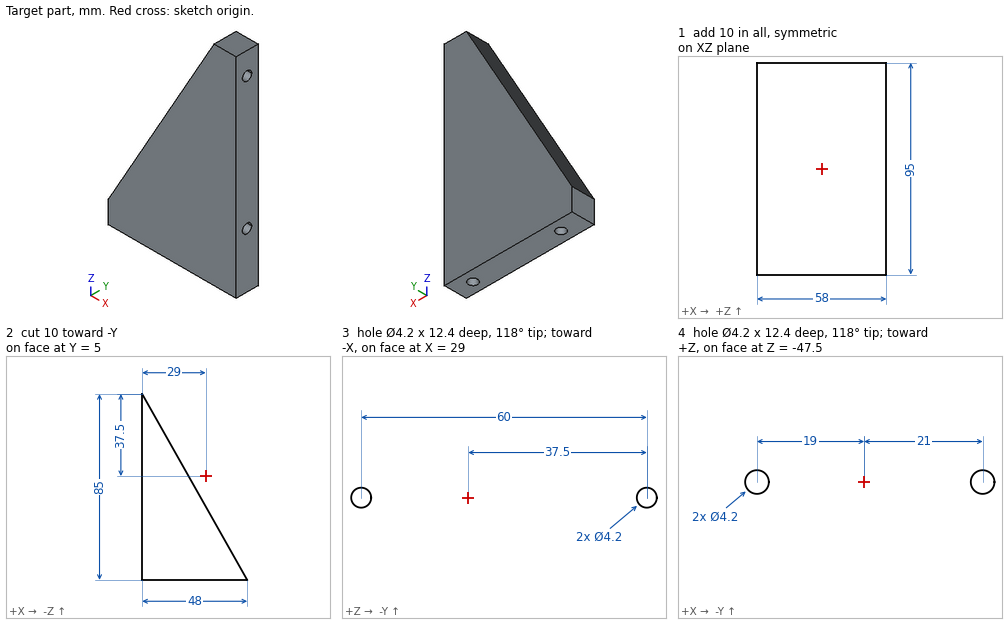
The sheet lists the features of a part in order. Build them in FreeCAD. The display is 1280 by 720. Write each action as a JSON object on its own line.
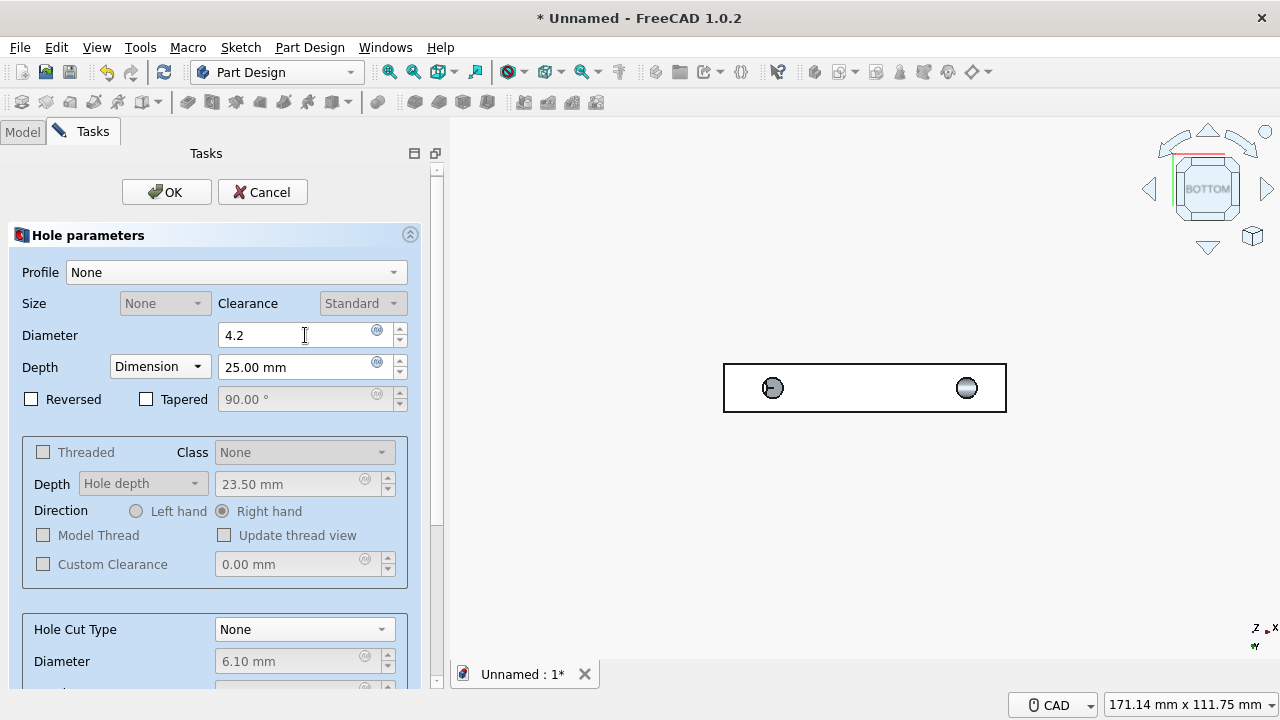
{"action": "triple_click", "coordinate": [305, 367]}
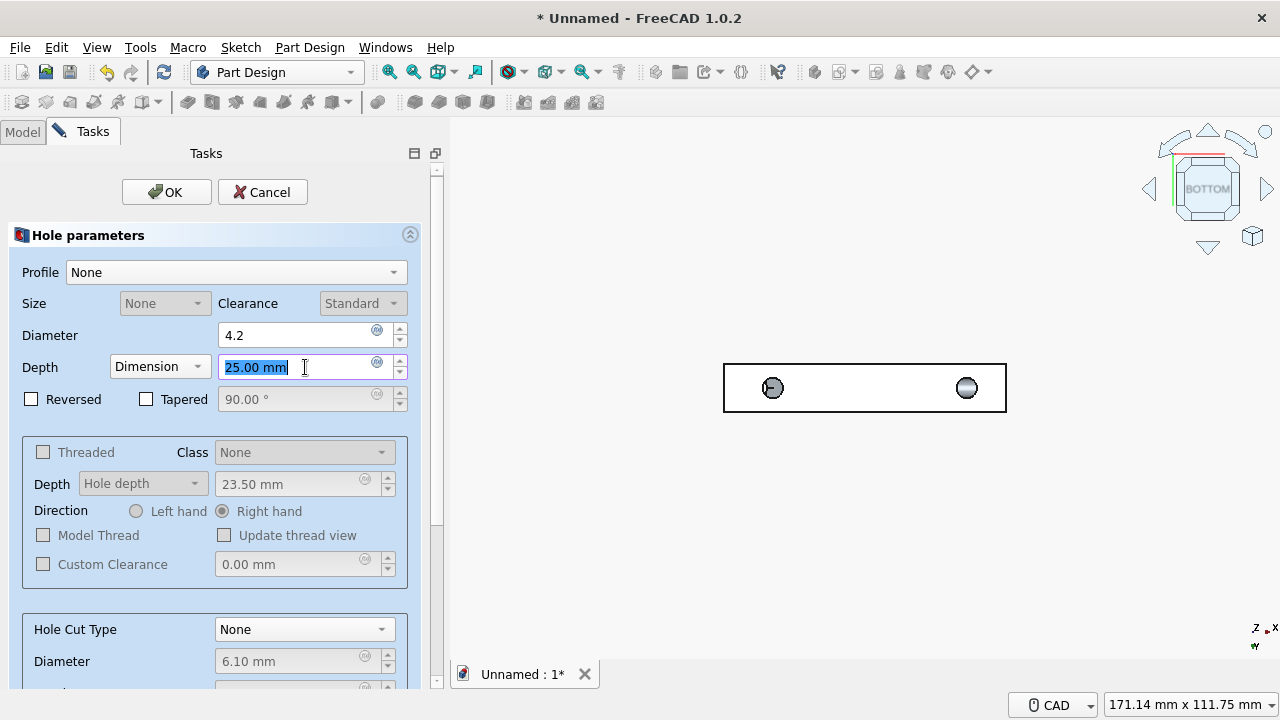
{"action": "type", "text": "12.4"}
{"action": "key", "text": "Tab"}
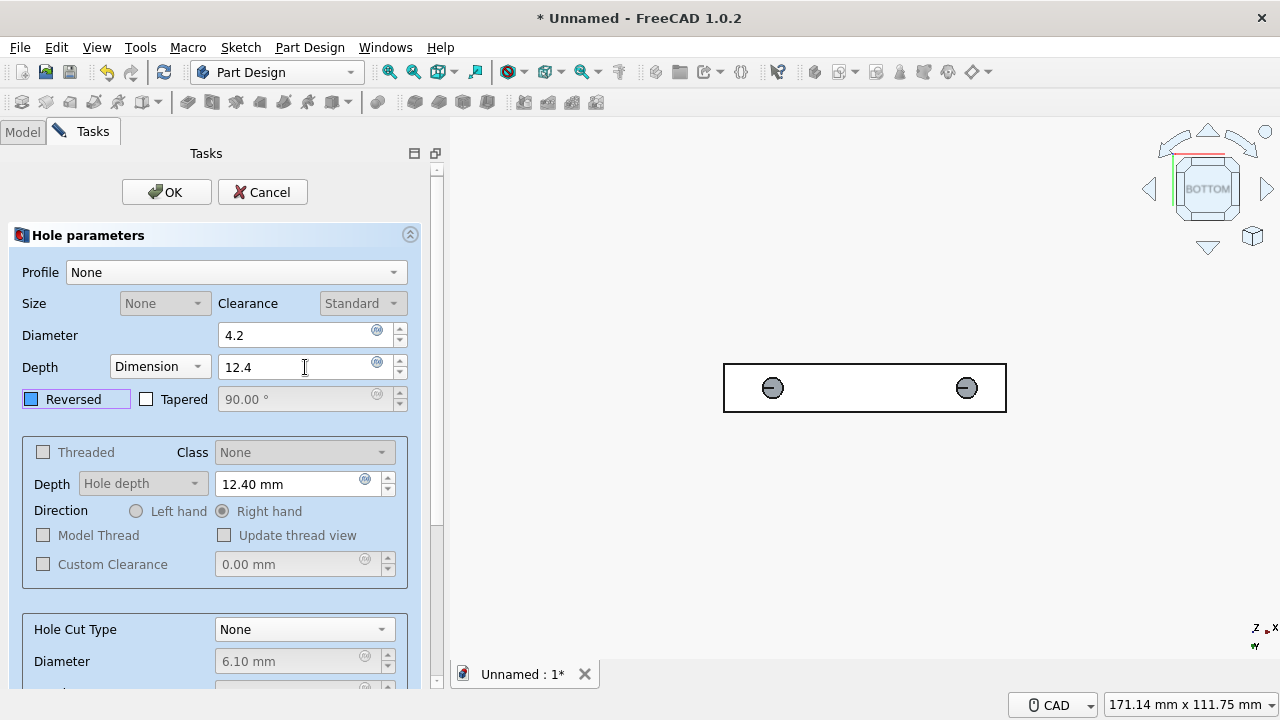
{"action": "left_click", "coordinate": [167, 192]}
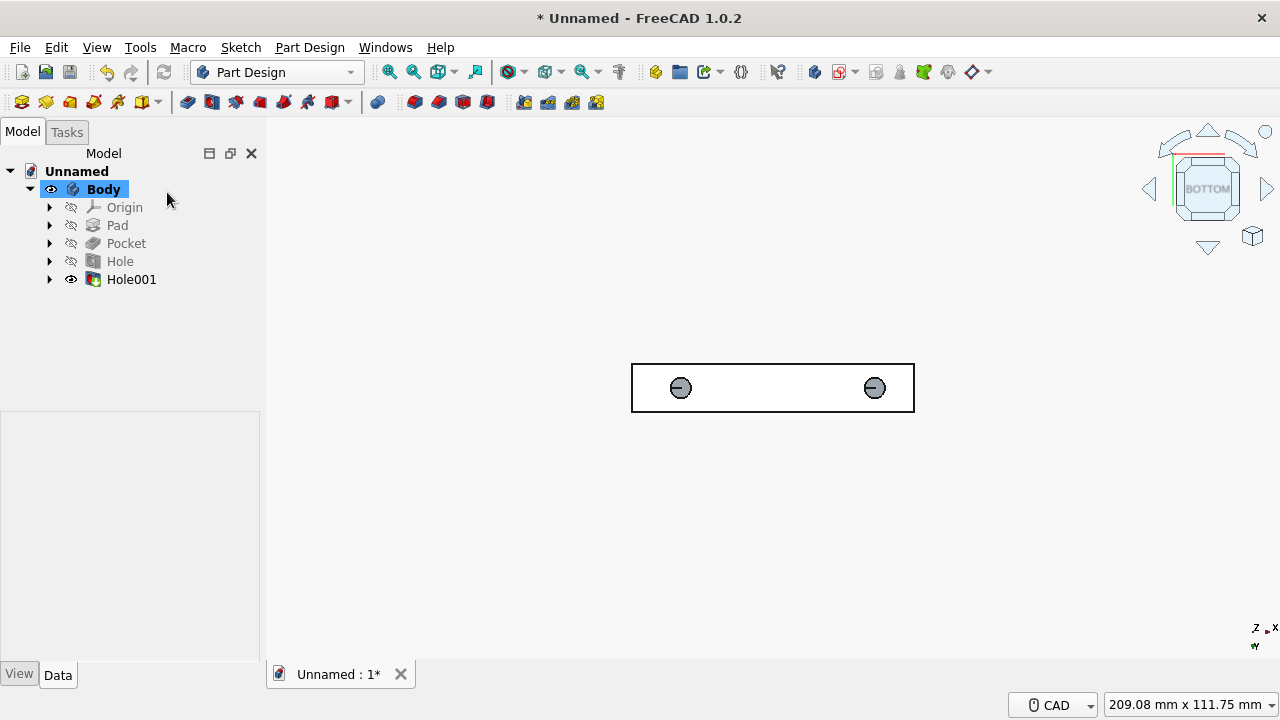
{"action": "key", "text": "0"}